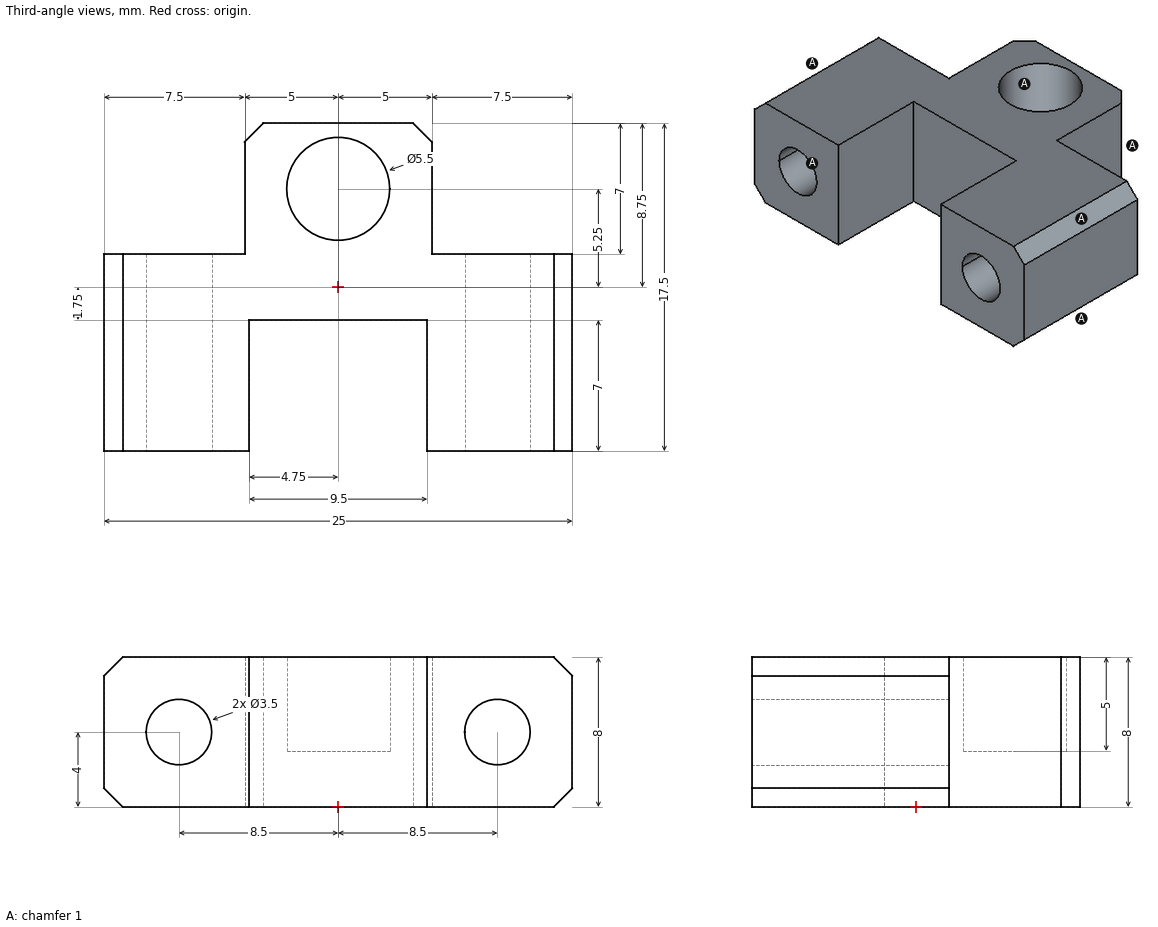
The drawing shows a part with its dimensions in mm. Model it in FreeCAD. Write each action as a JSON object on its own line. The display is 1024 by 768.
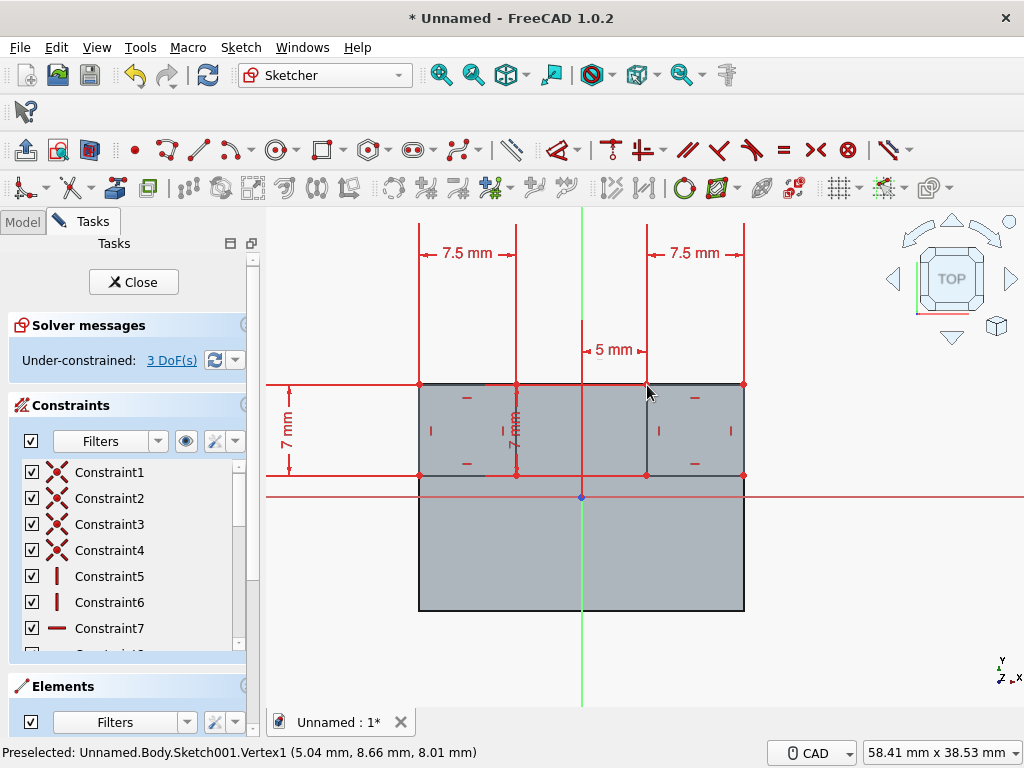
{"action": "left_click", "coordinate": [516, 476]}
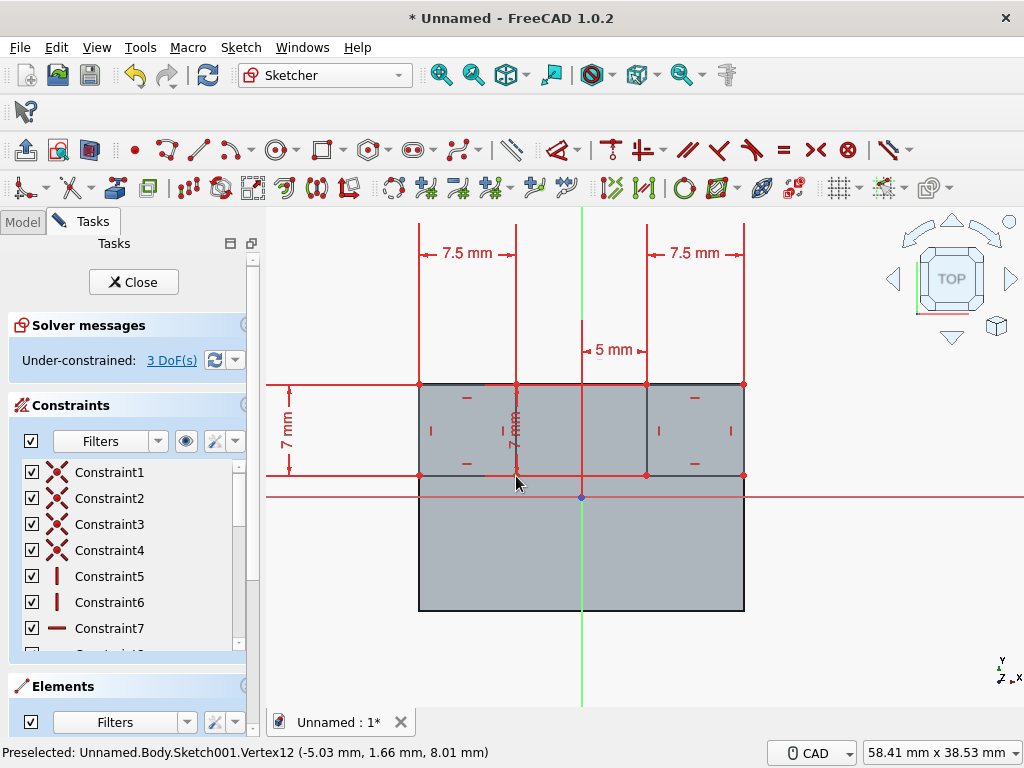
{"action": "key", "text": "l"}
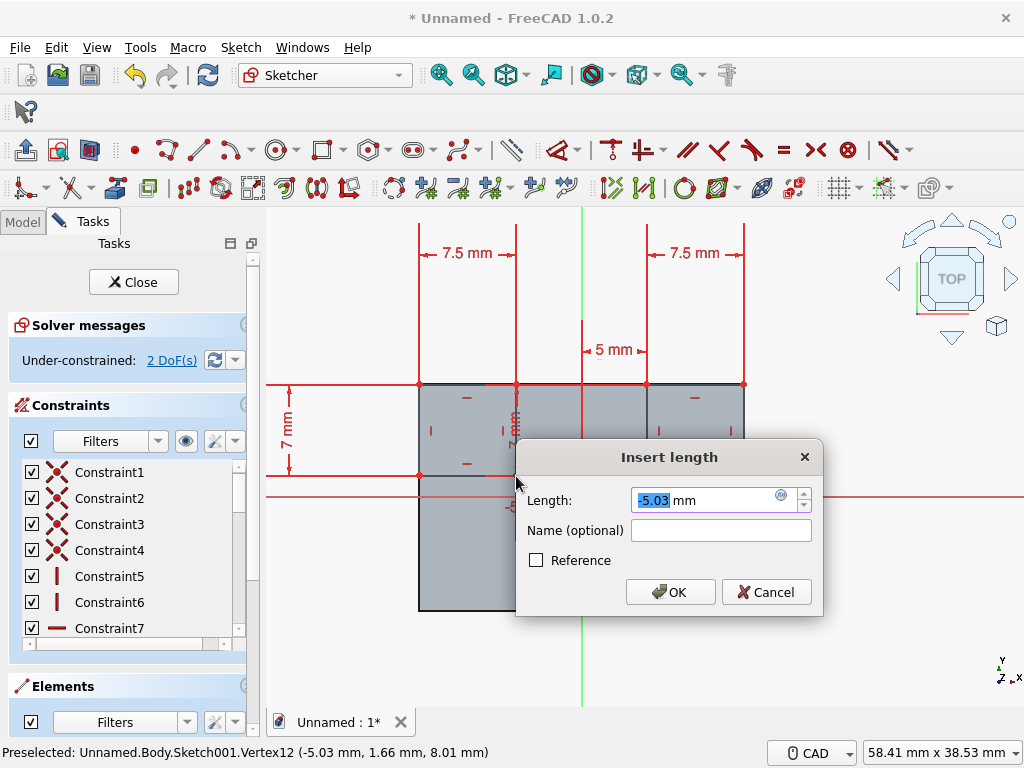
{"action": "type", "text": "-5"}
{"action": "key", "text": "Return"}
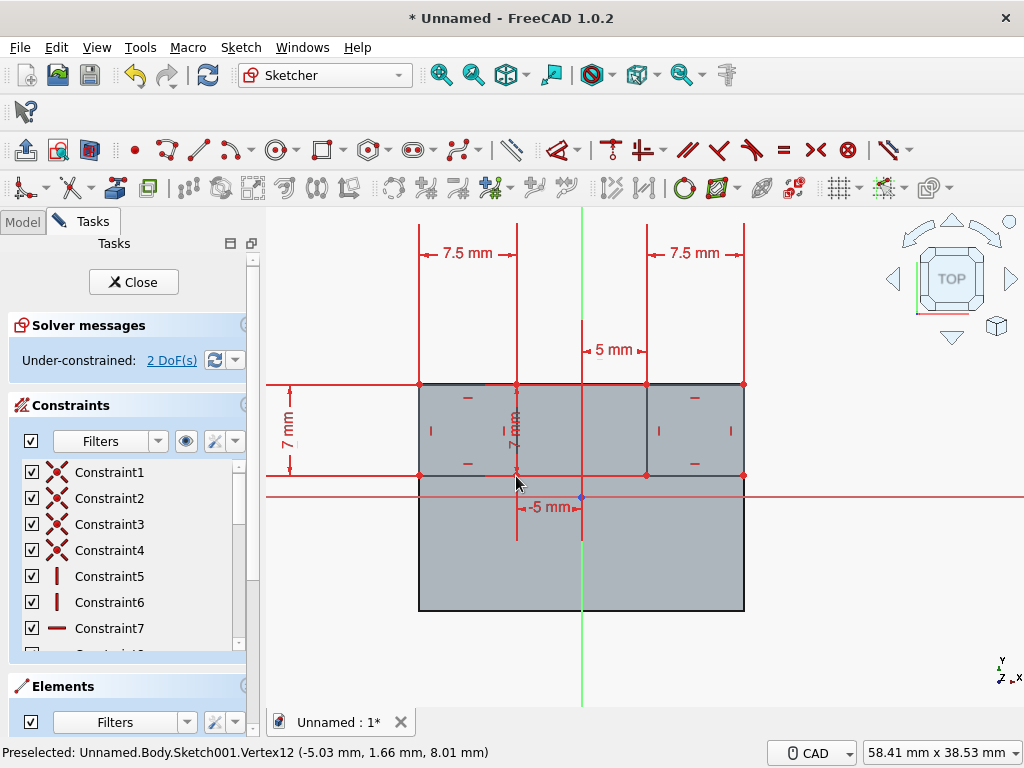
{"action": "left_click", "coordinate": [647, 385]}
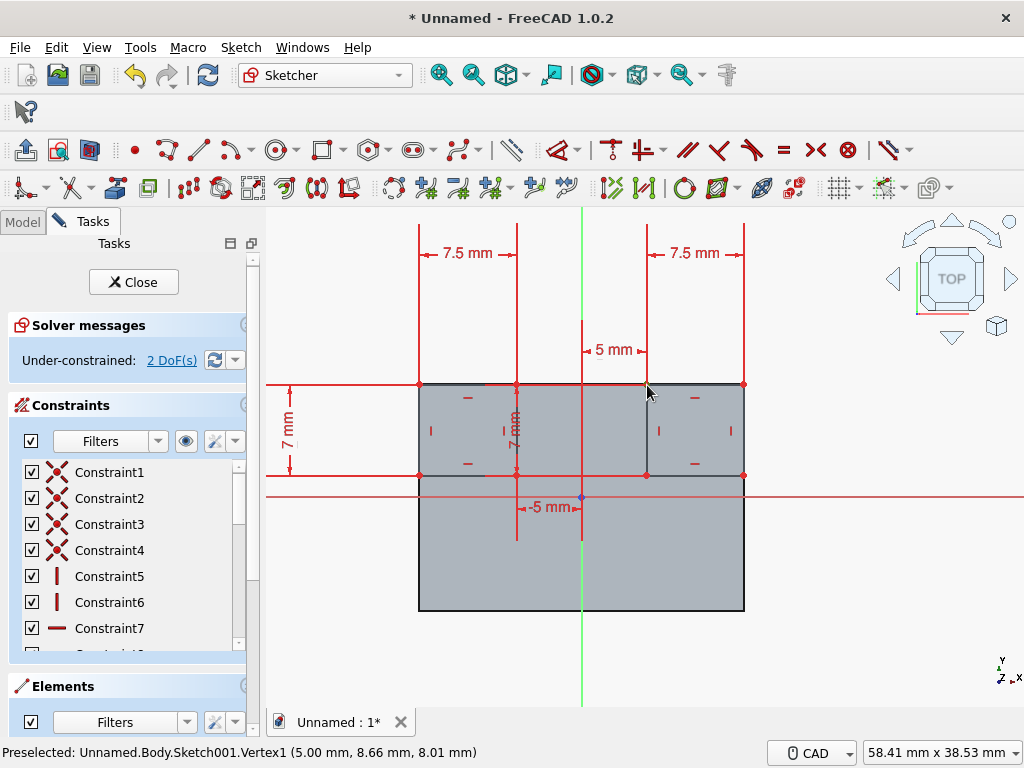
{"action": "key", "text": "i"}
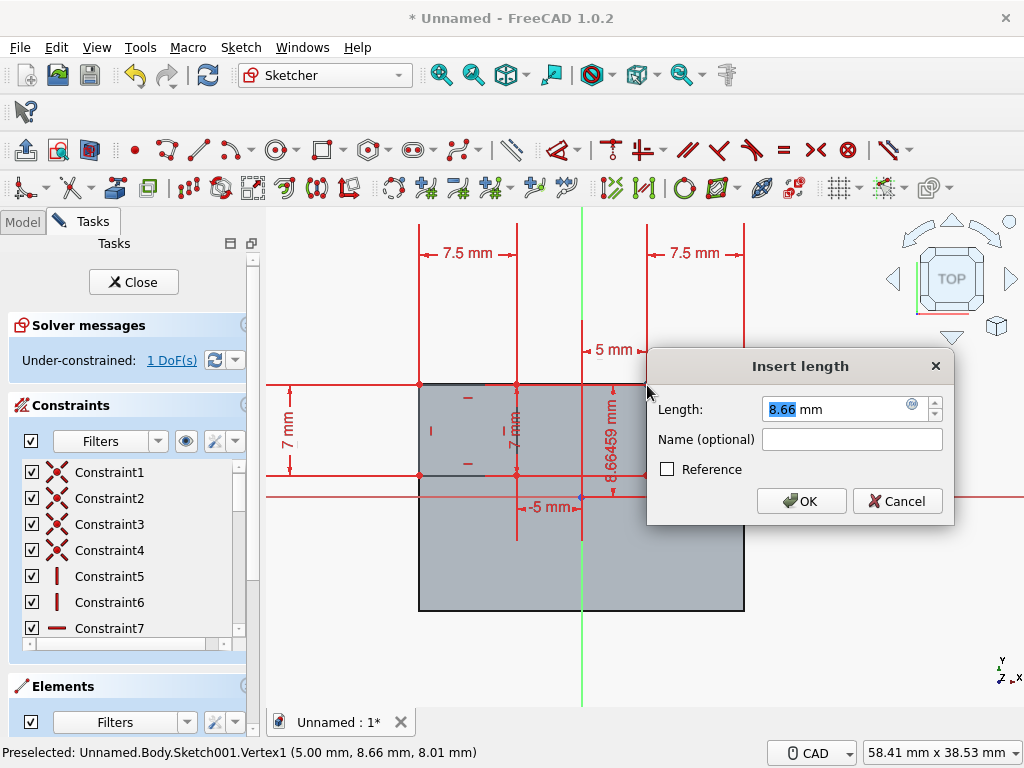
{"action": "type", "text": "8.75"}
{"action": "key", "text": "Return"}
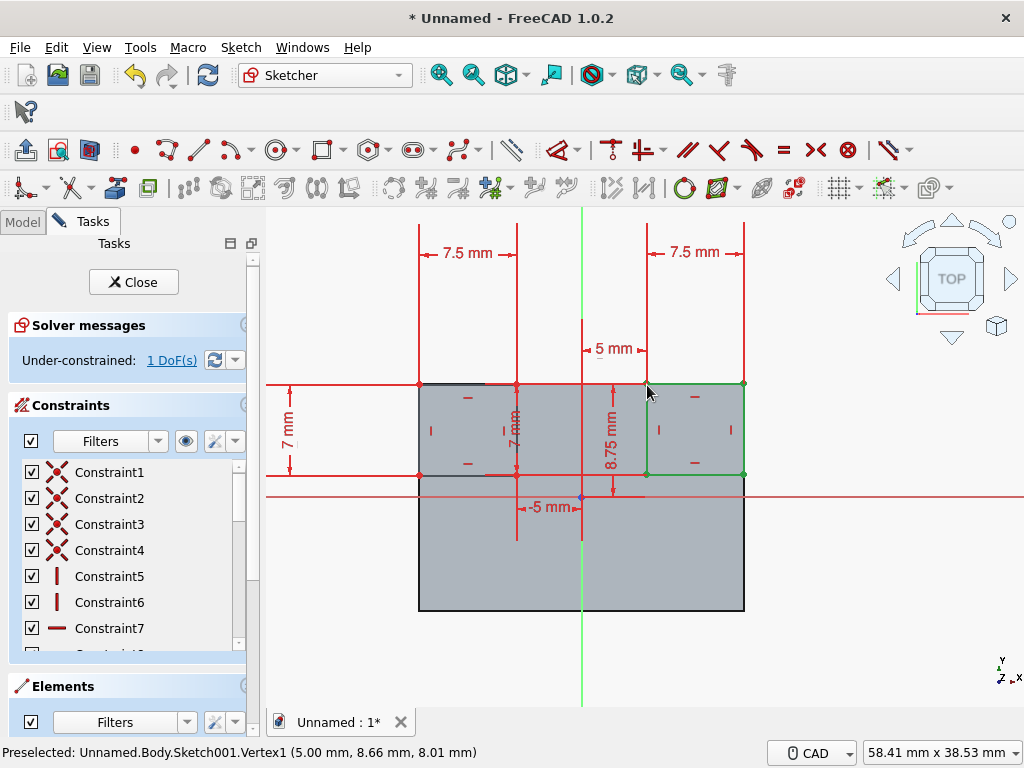
{"action": "left_click", "coordinate": [419, 385]}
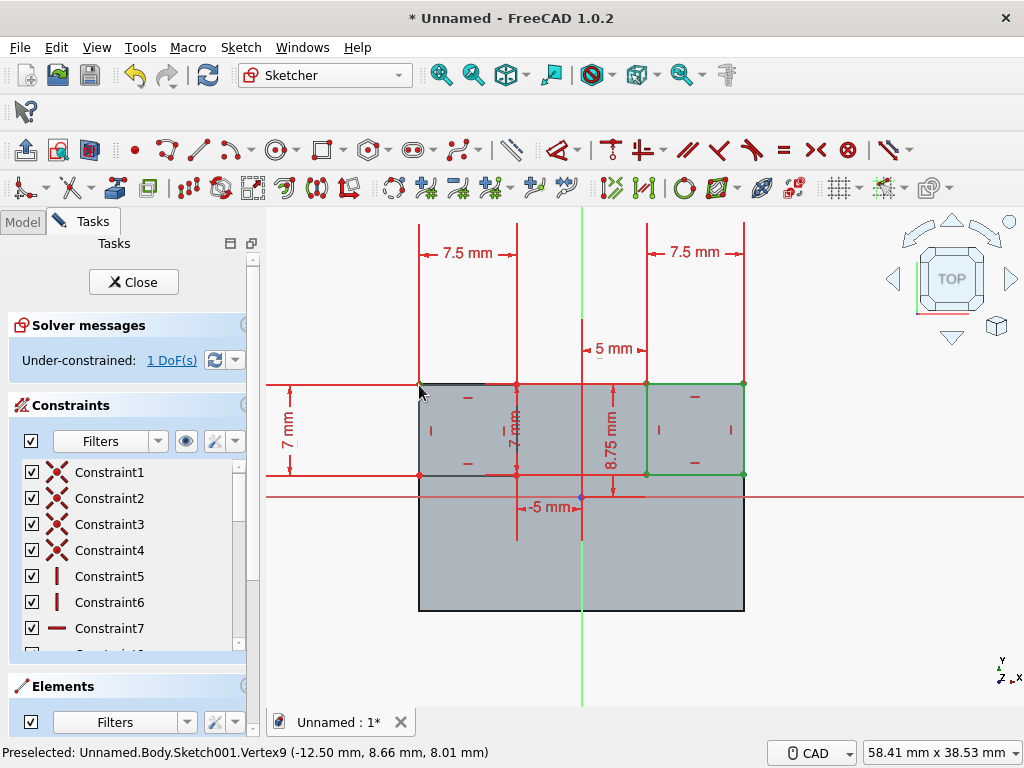
{"action": "left_click", "coordinate": [580, 150]}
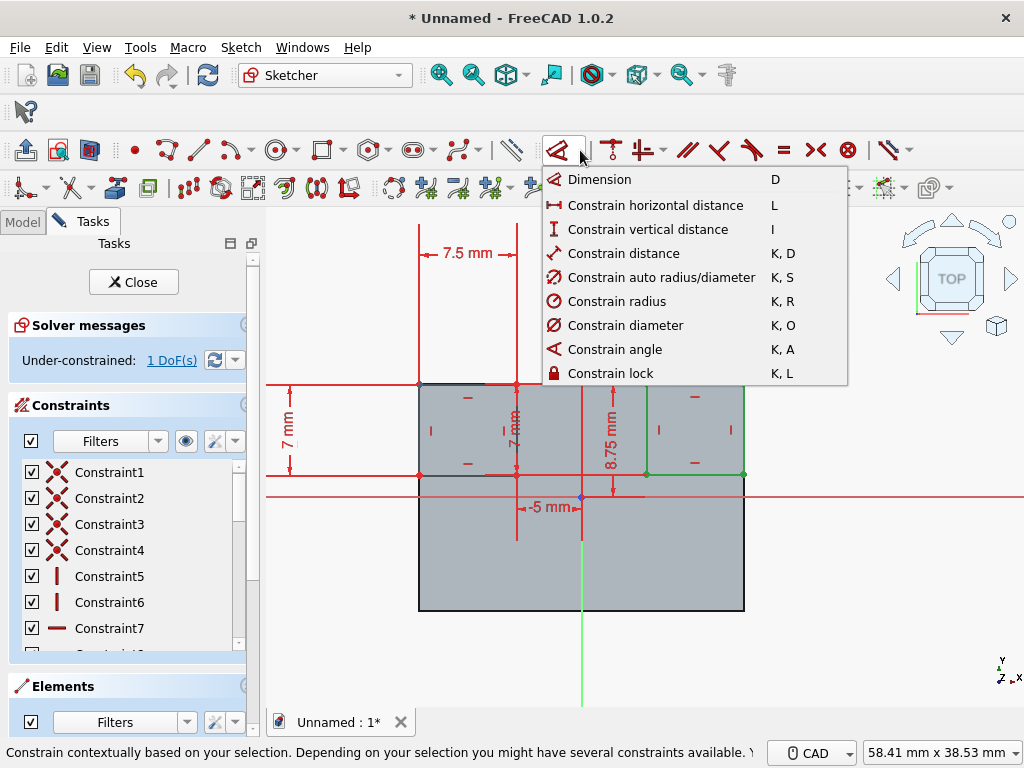
{"action": "left_click", "coordinate": [695, 229]}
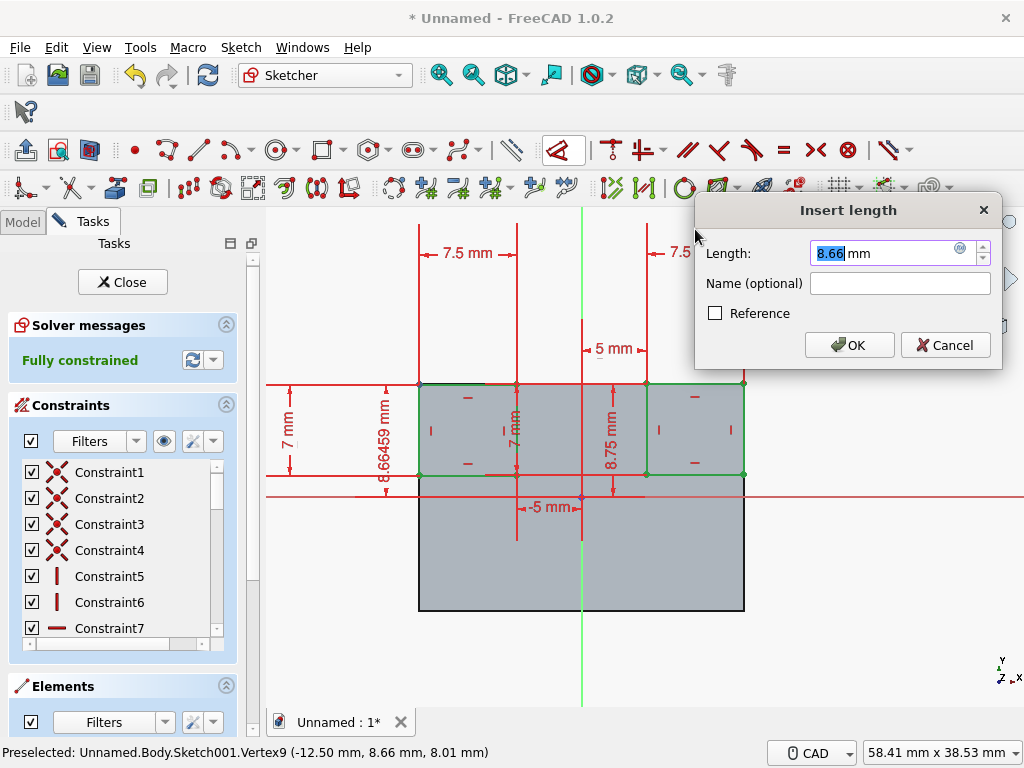
{"action": "type", "text": "8.75"}
{"action": "key", "text": "Return"}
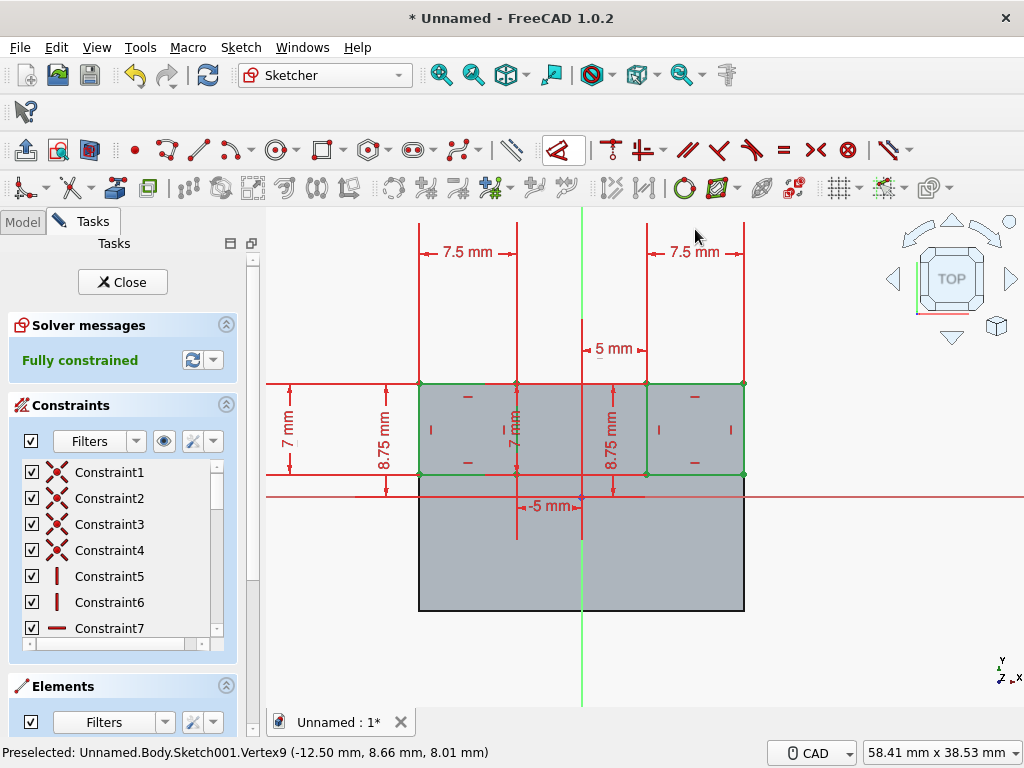
{"action": "left_click", "coordinate": [123, 282]}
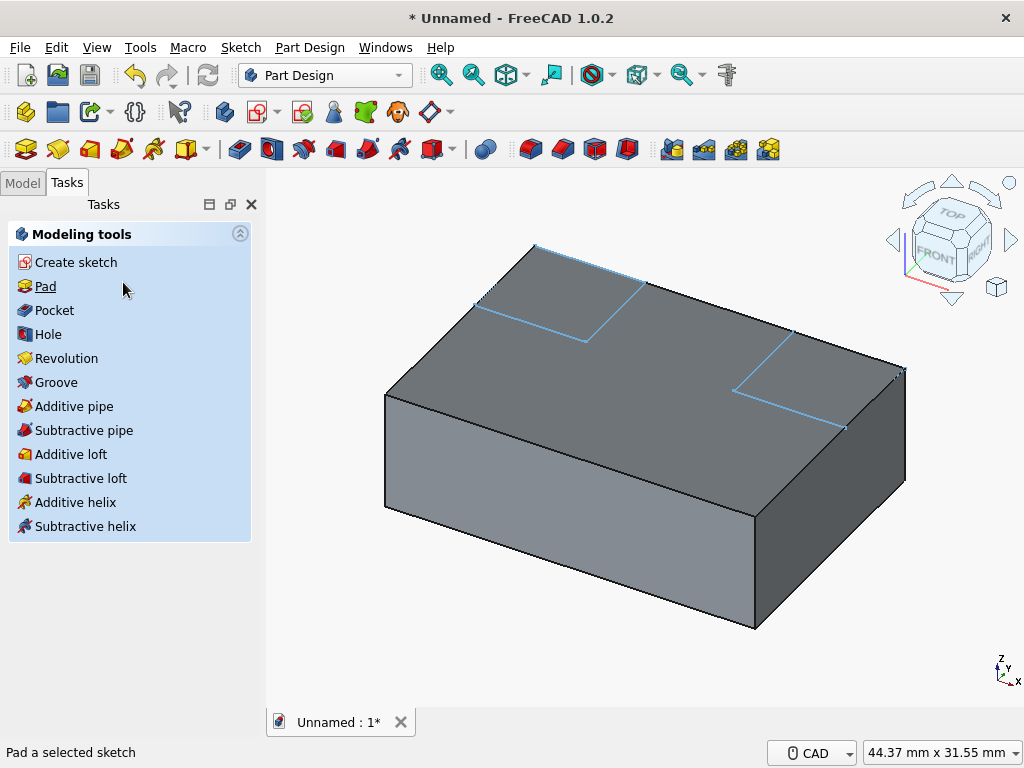
{"action": "left_click", "coordinate": [240, 150]}